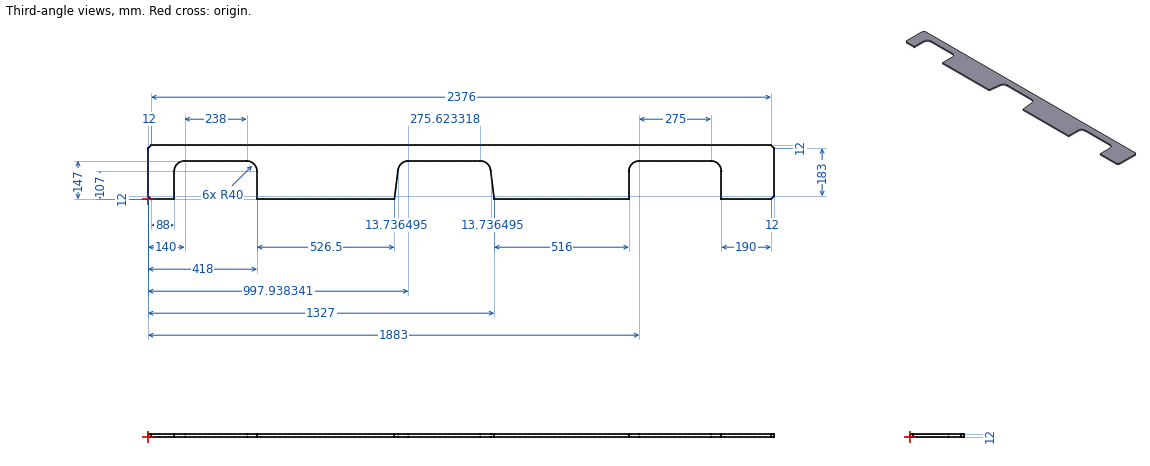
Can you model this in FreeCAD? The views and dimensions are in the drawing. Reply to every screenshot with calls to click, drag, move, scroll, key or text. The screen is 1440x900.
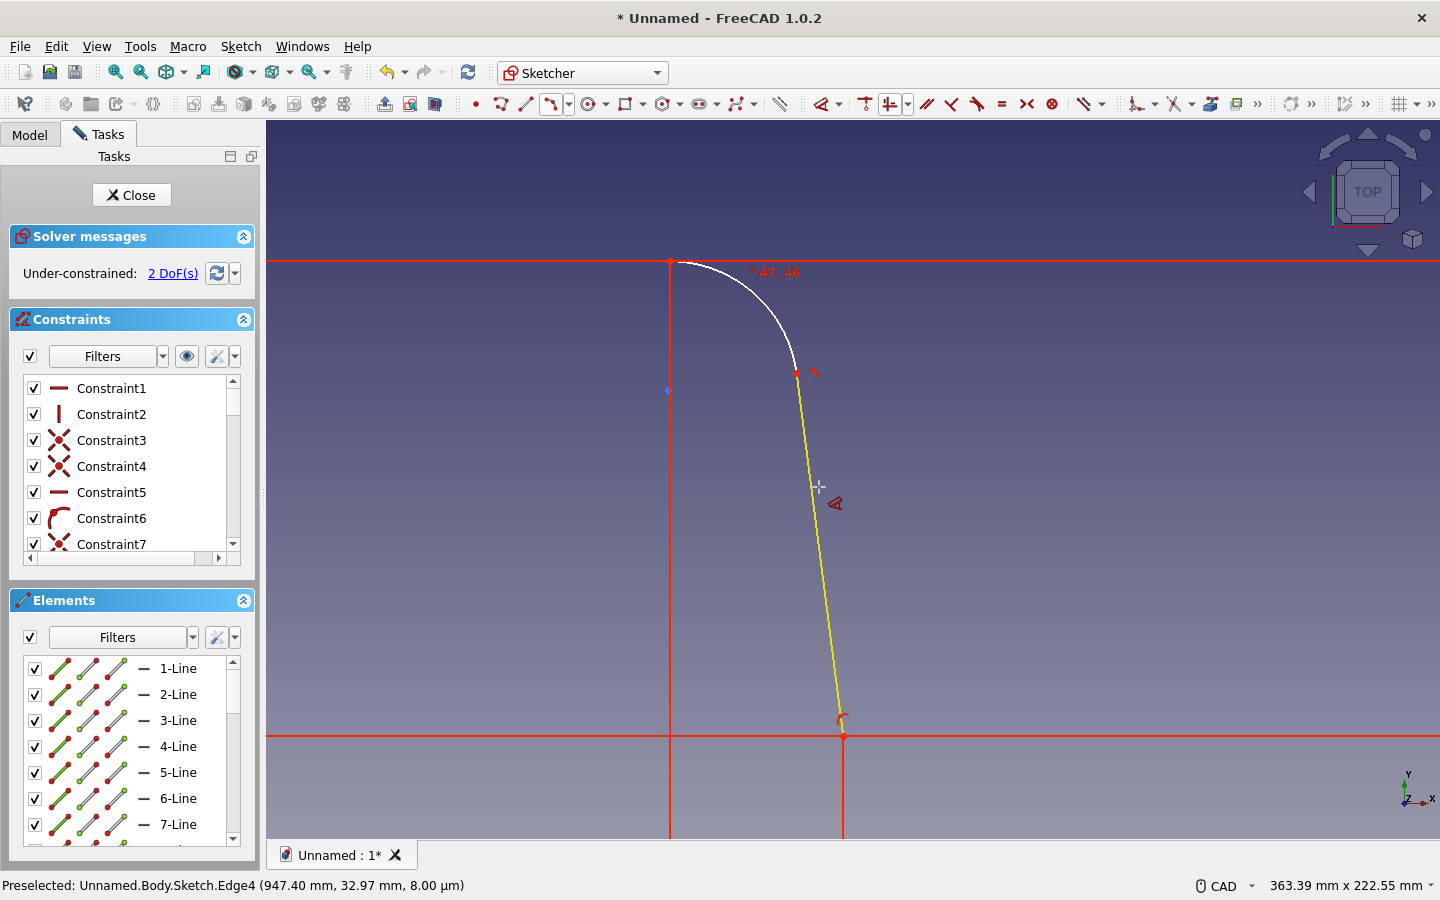
click(811, 482)
click(820, 770)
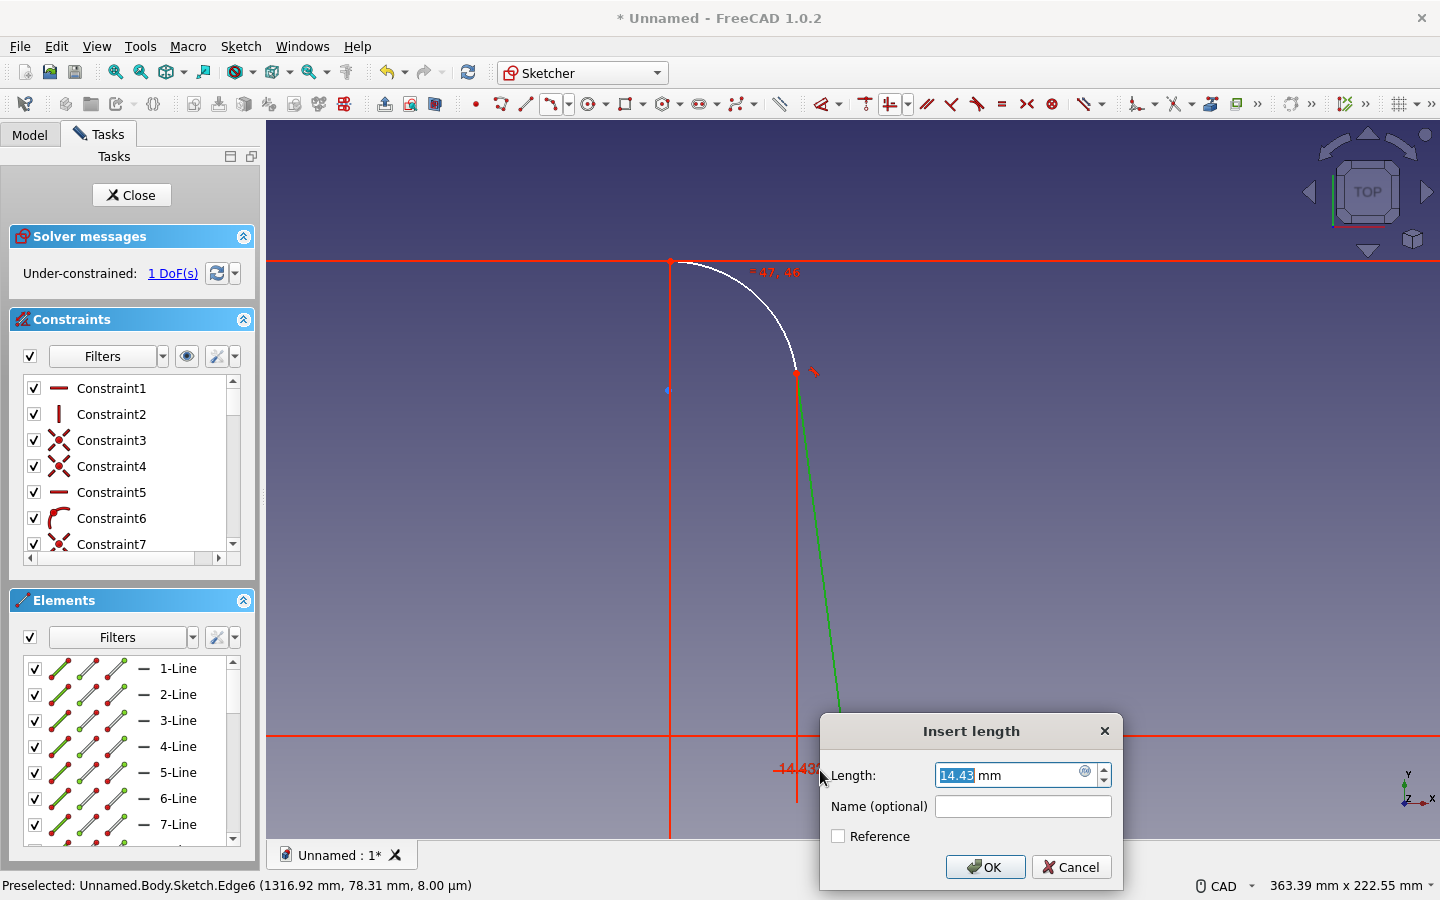
text(13.736495)
key(Return)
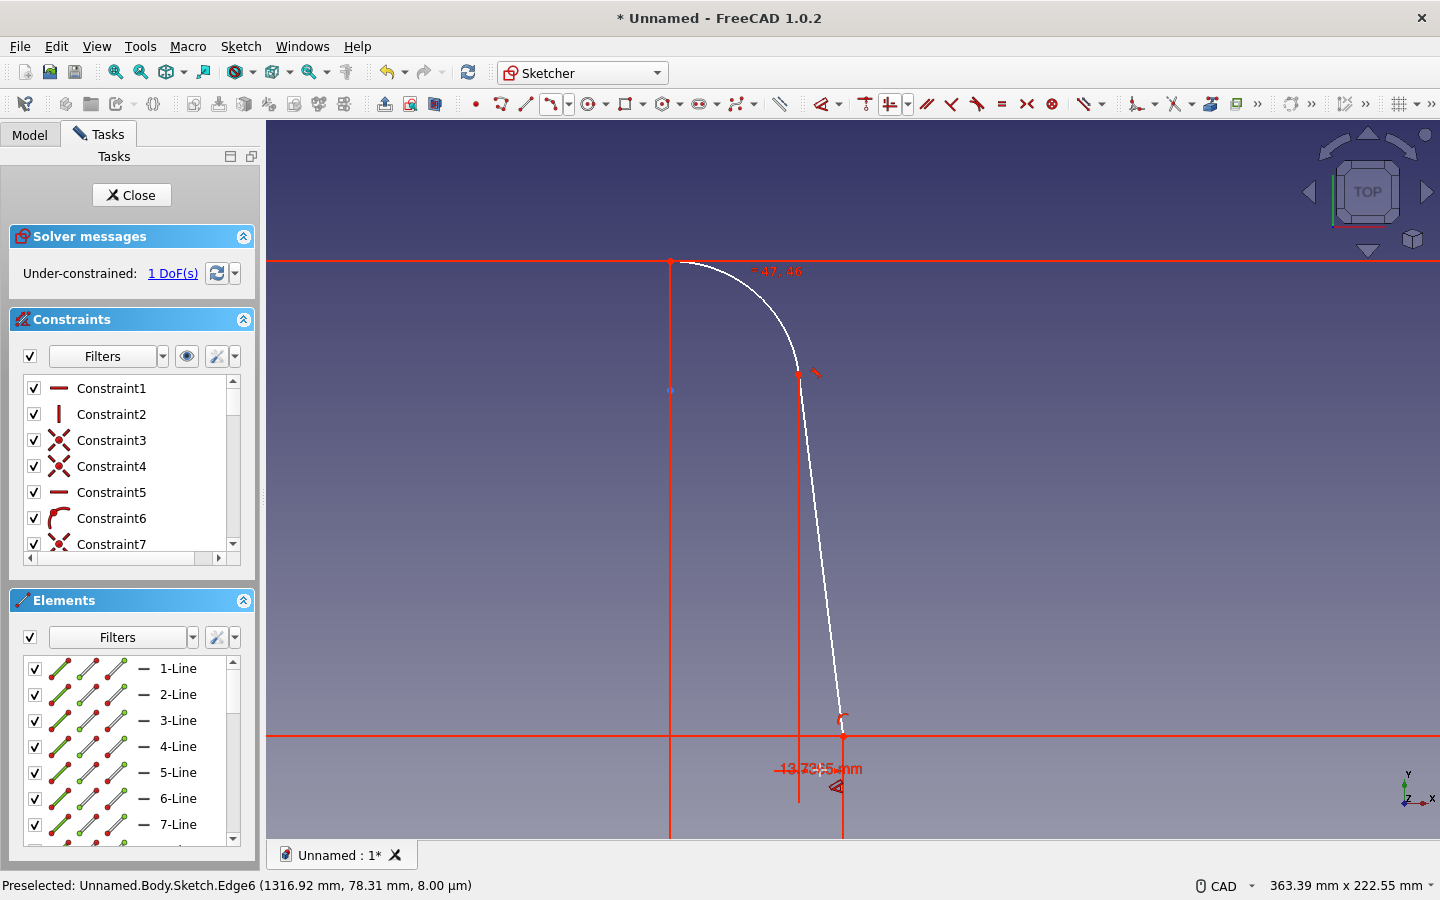
scroll(820, 487, down, 12)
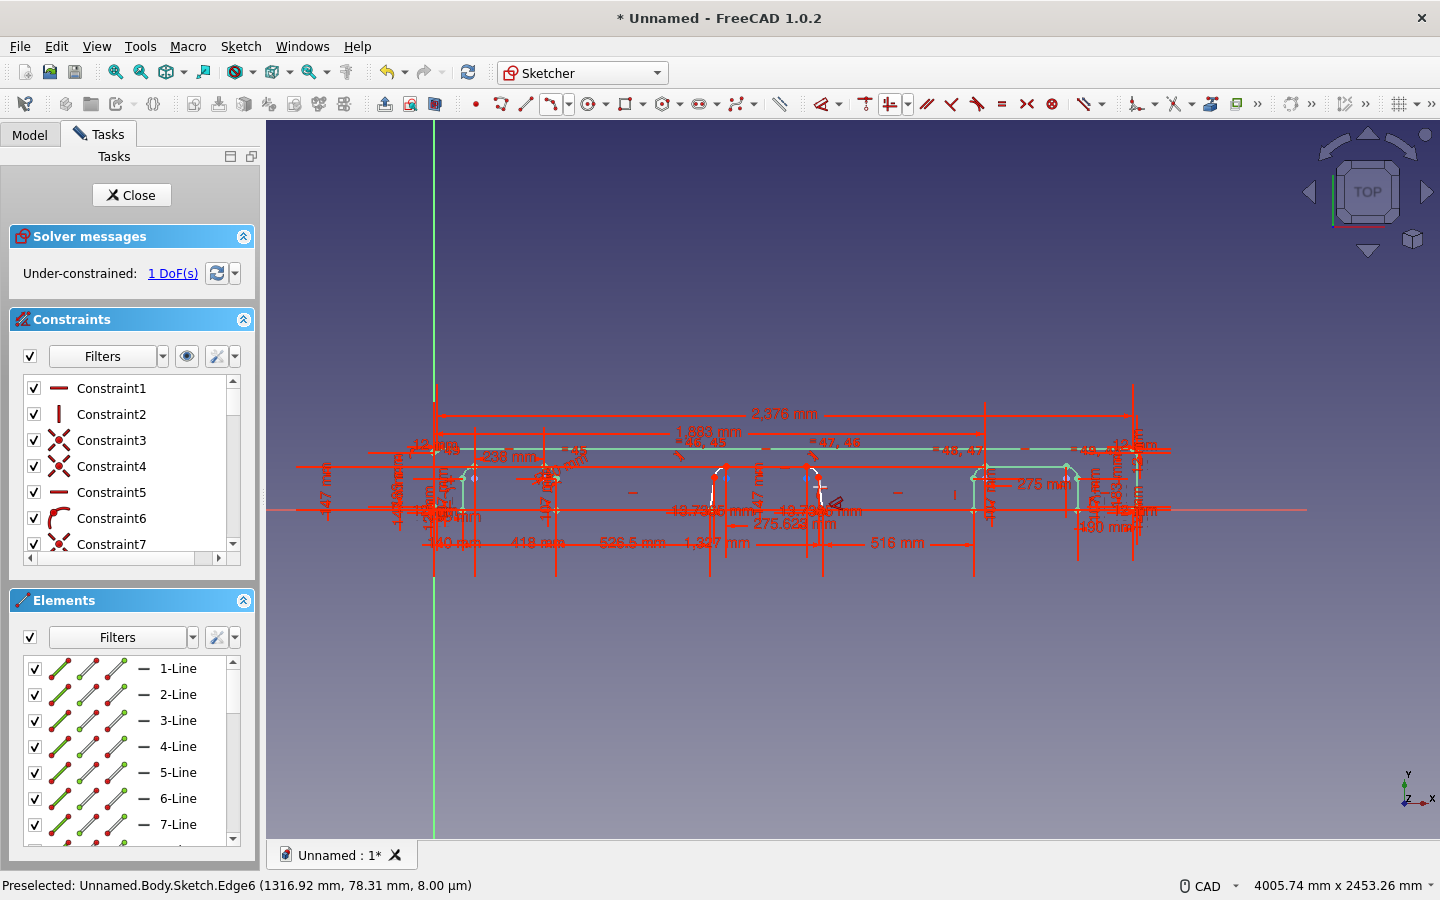
click(726, 467)
click(580, 433)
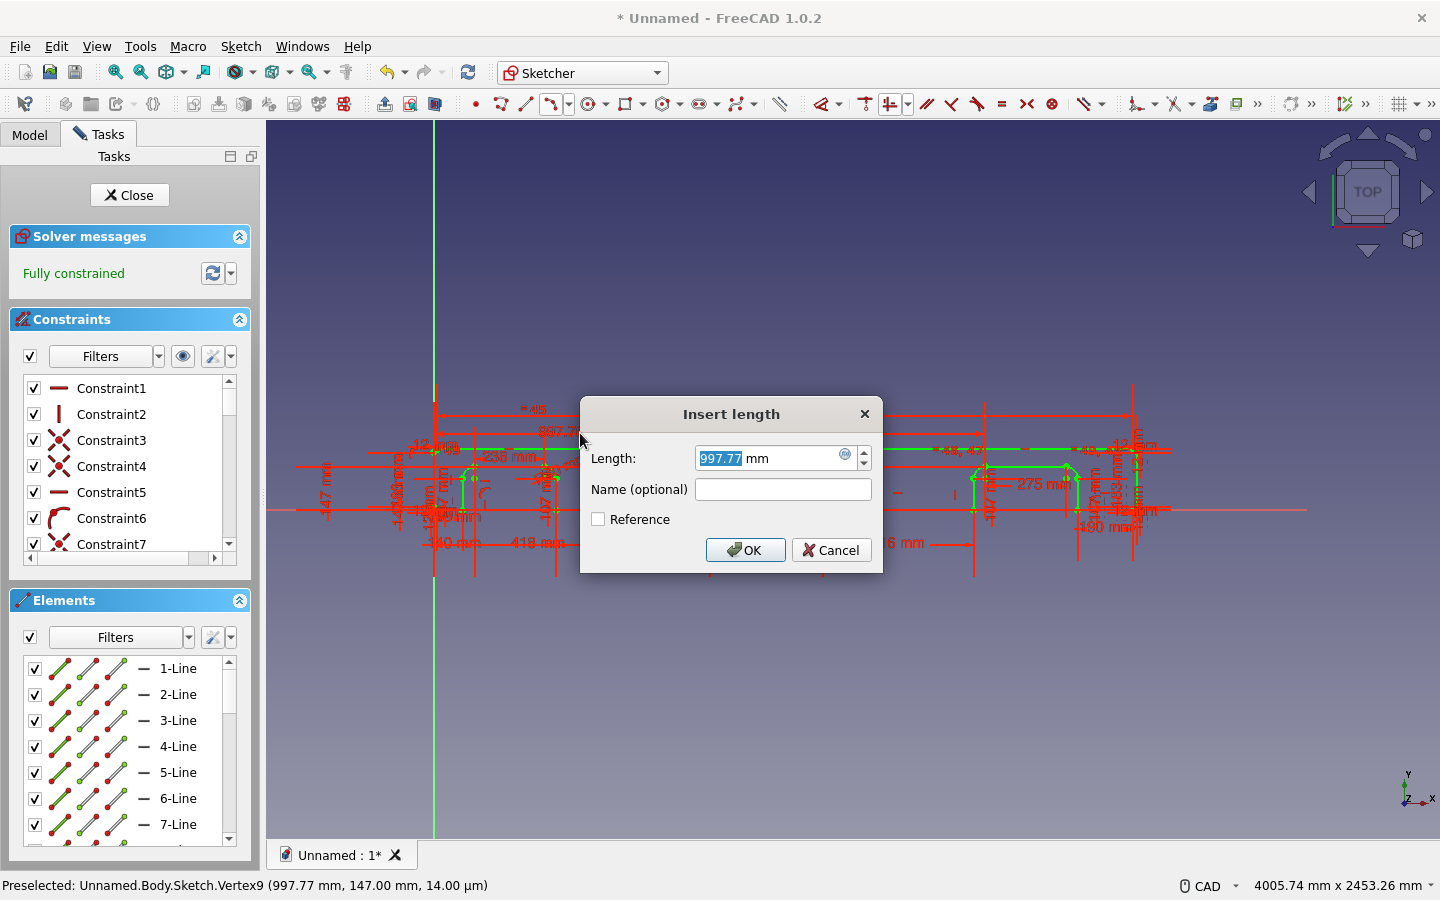
text(997.938341)
key(Return)
key(Escape)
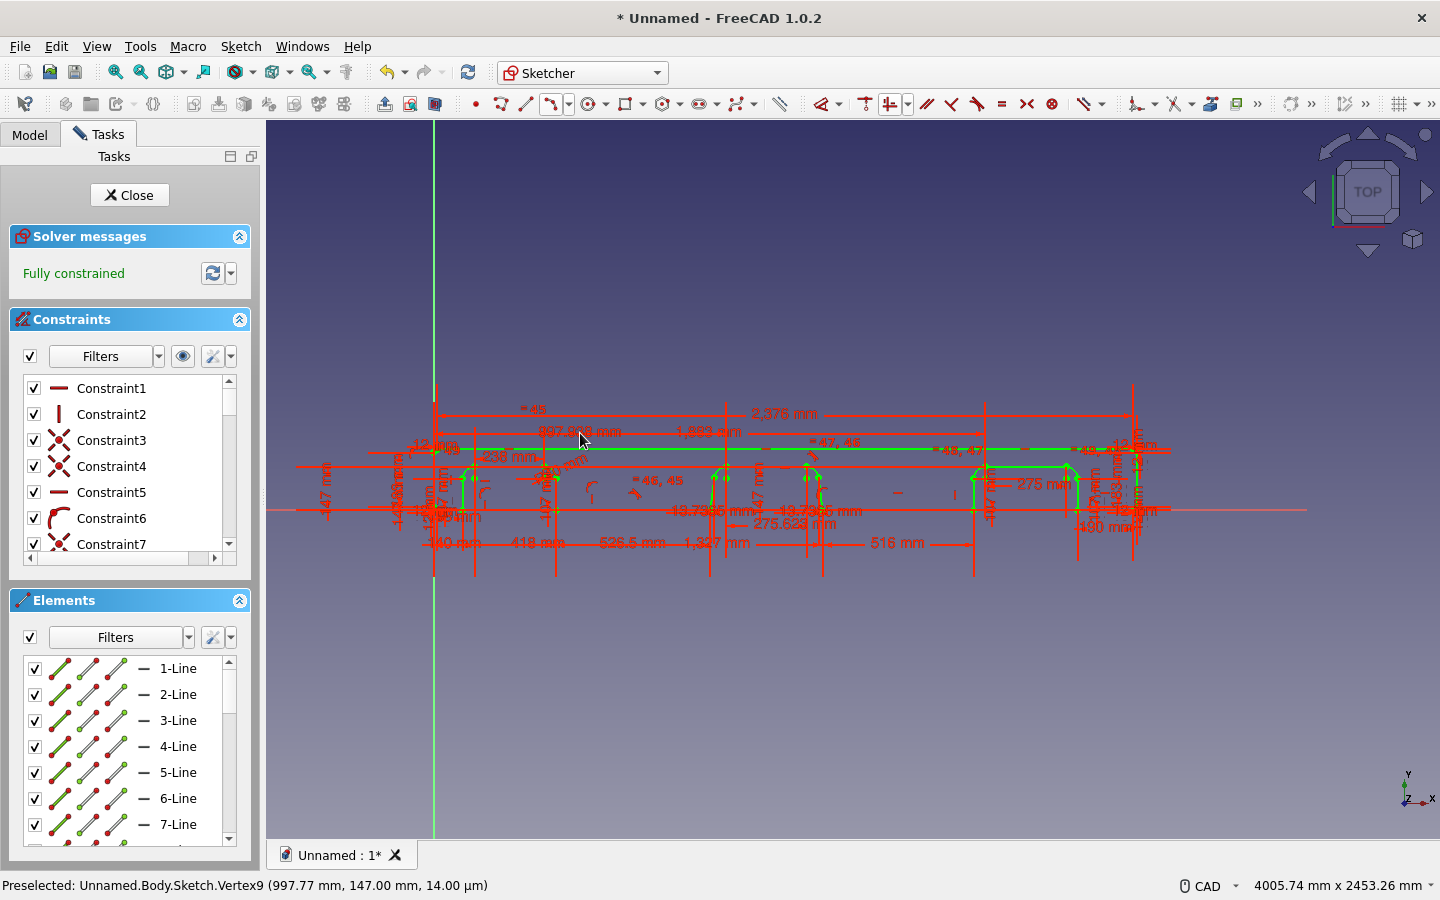
click(130, 195)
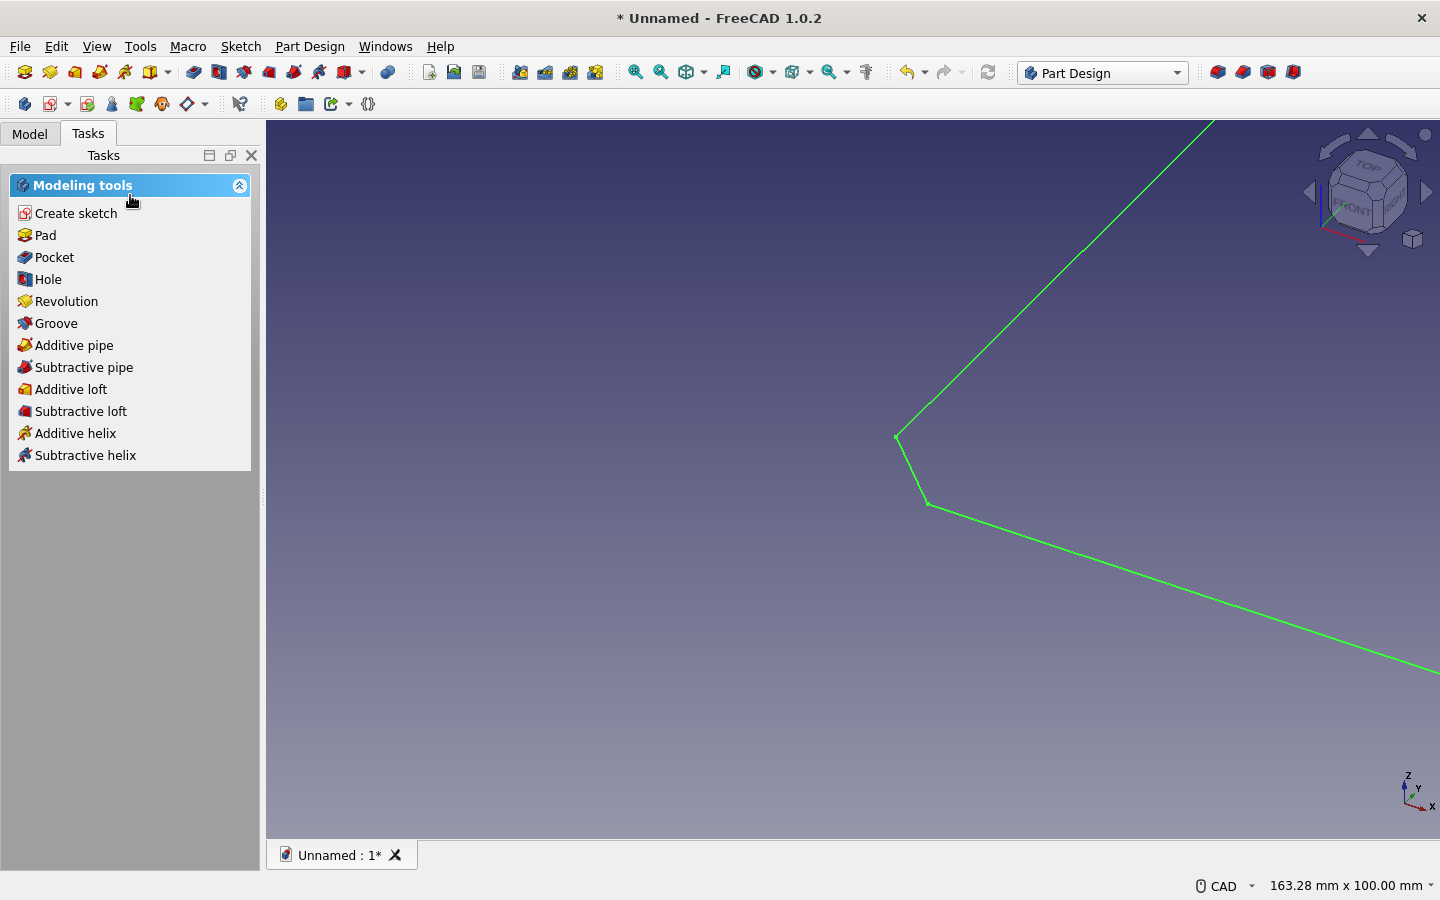
click(25, 72)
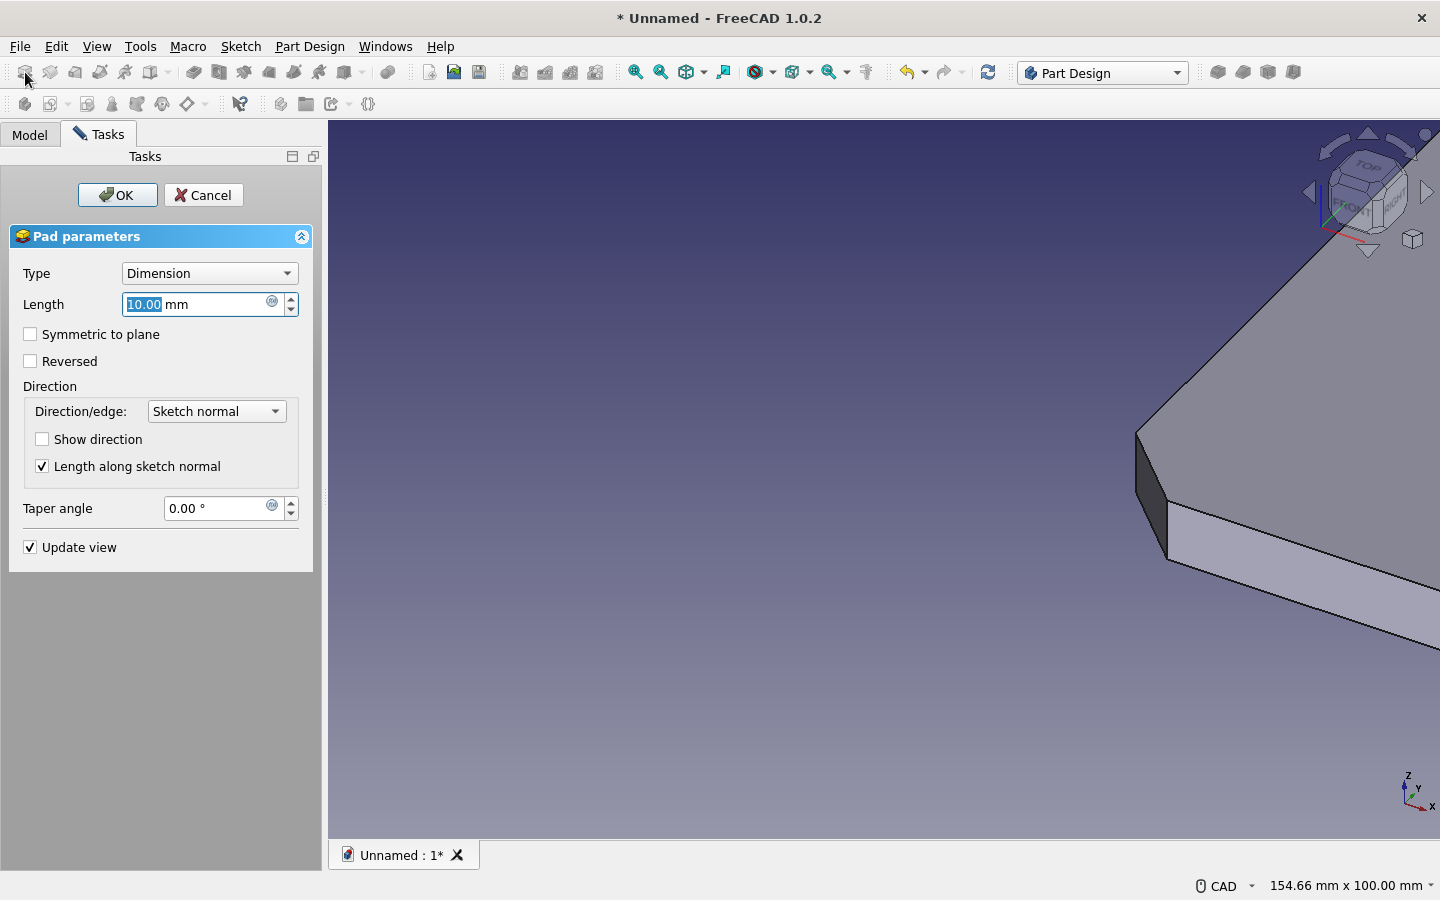
text(12)
key(Tab)